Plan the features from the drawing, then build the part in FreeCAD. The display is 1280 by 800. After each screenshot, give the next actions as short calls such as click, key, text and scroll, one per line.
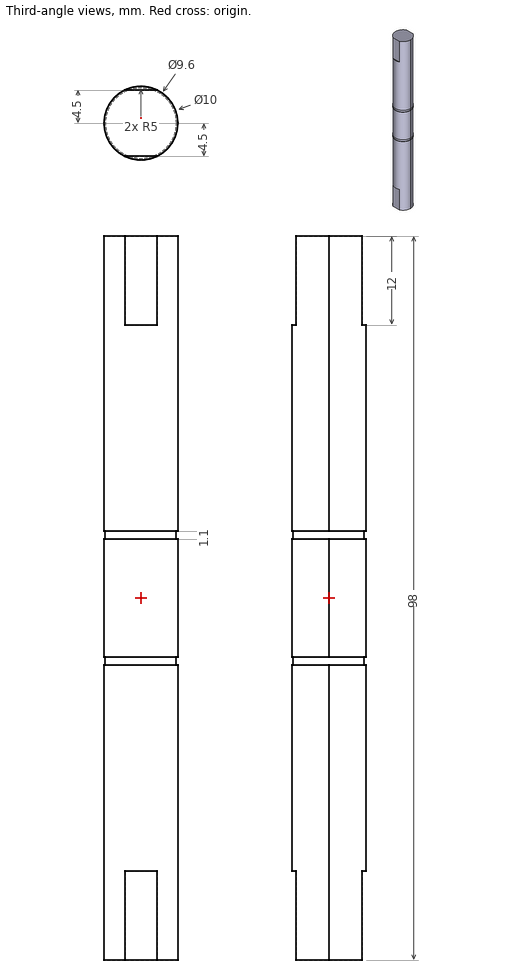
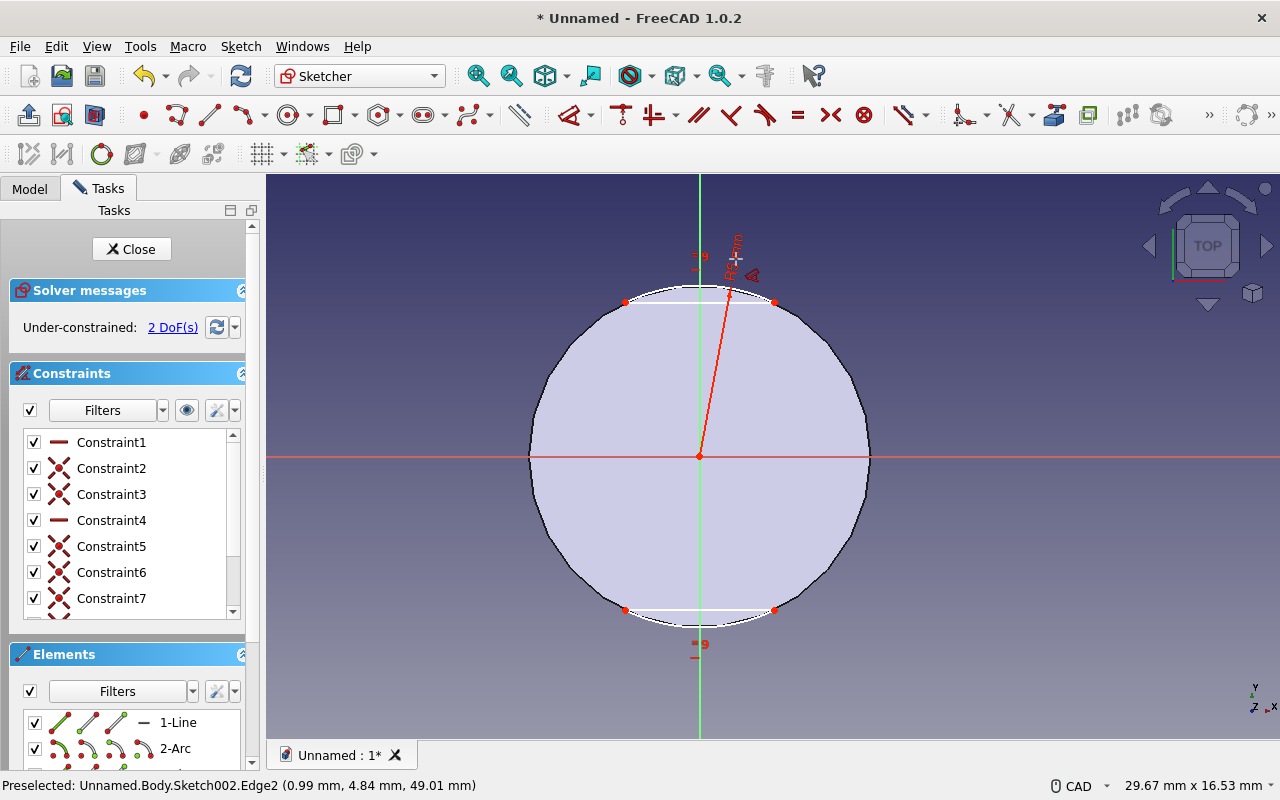
click(625, 303)
click(591, 380)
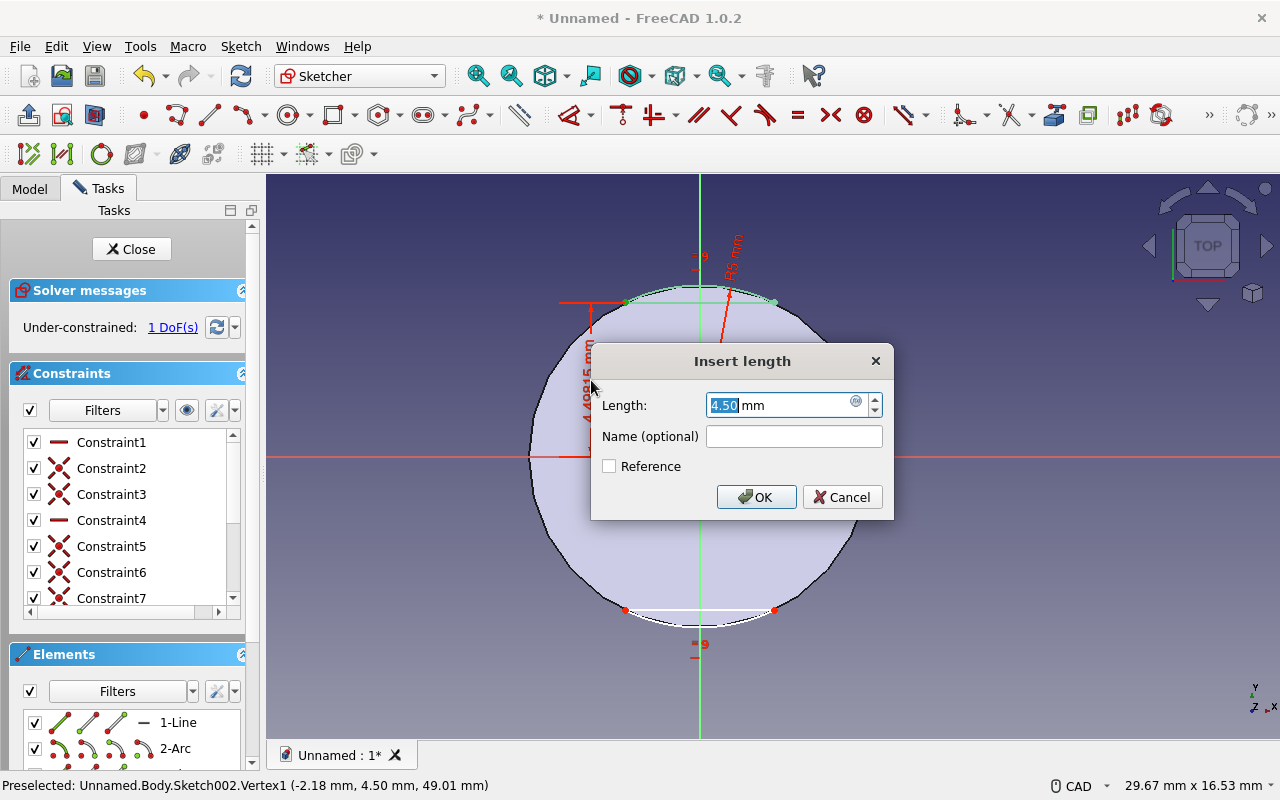
text(4.5)
key(Return)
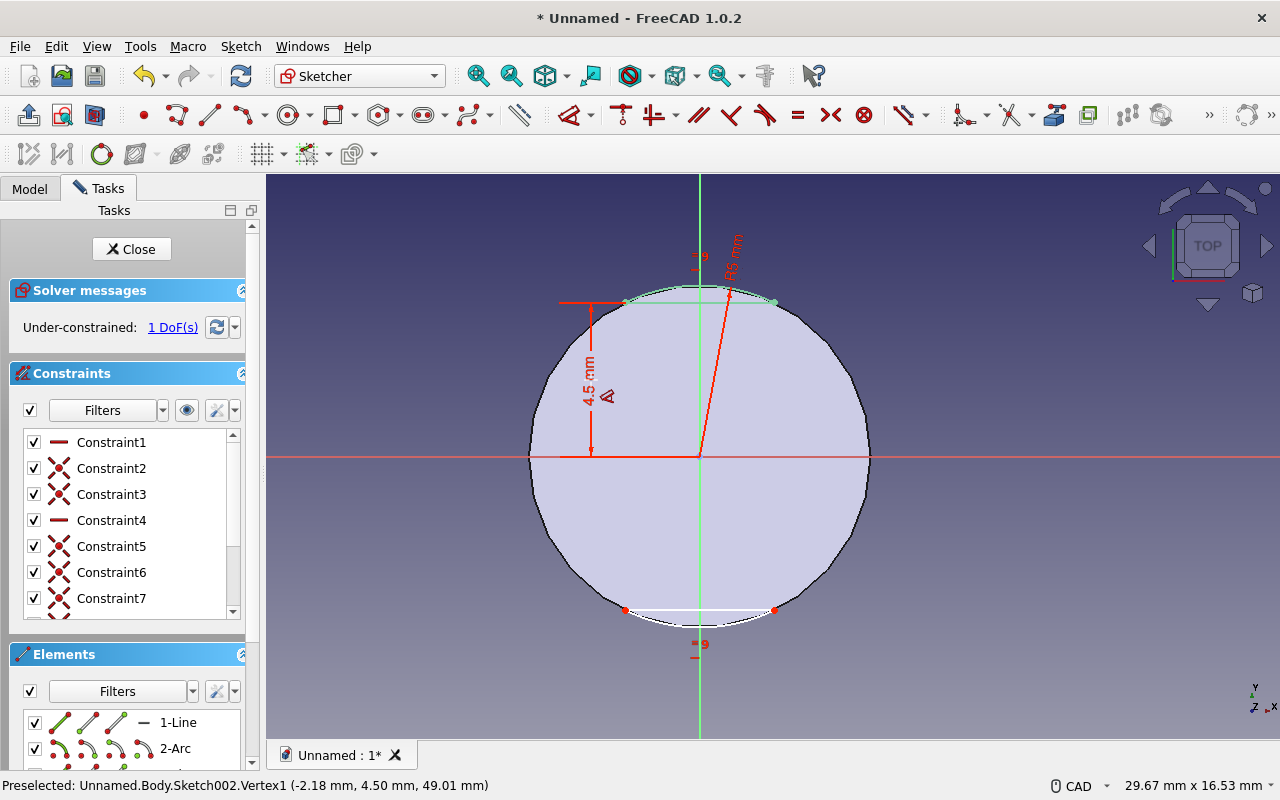
click(774, 610)
click(808, 533)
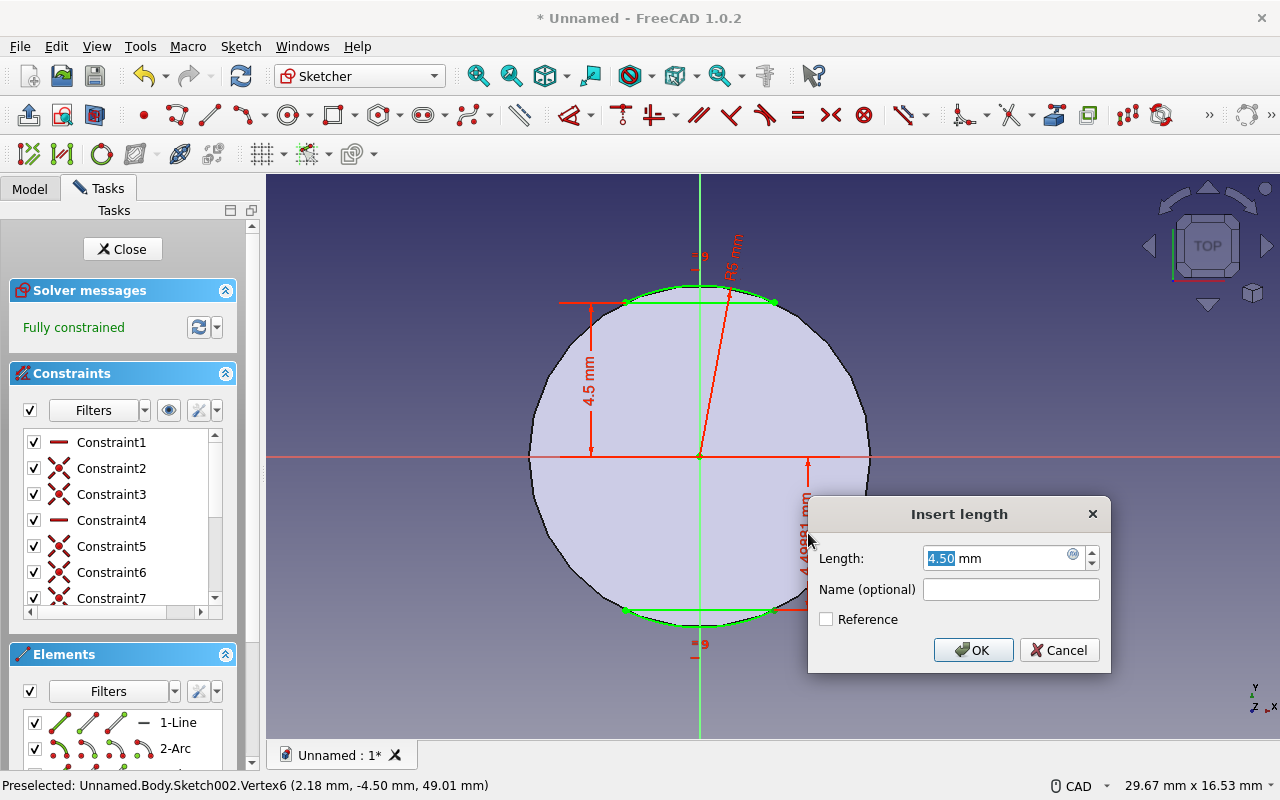
text(4.5)
key(Return)
key(Escape)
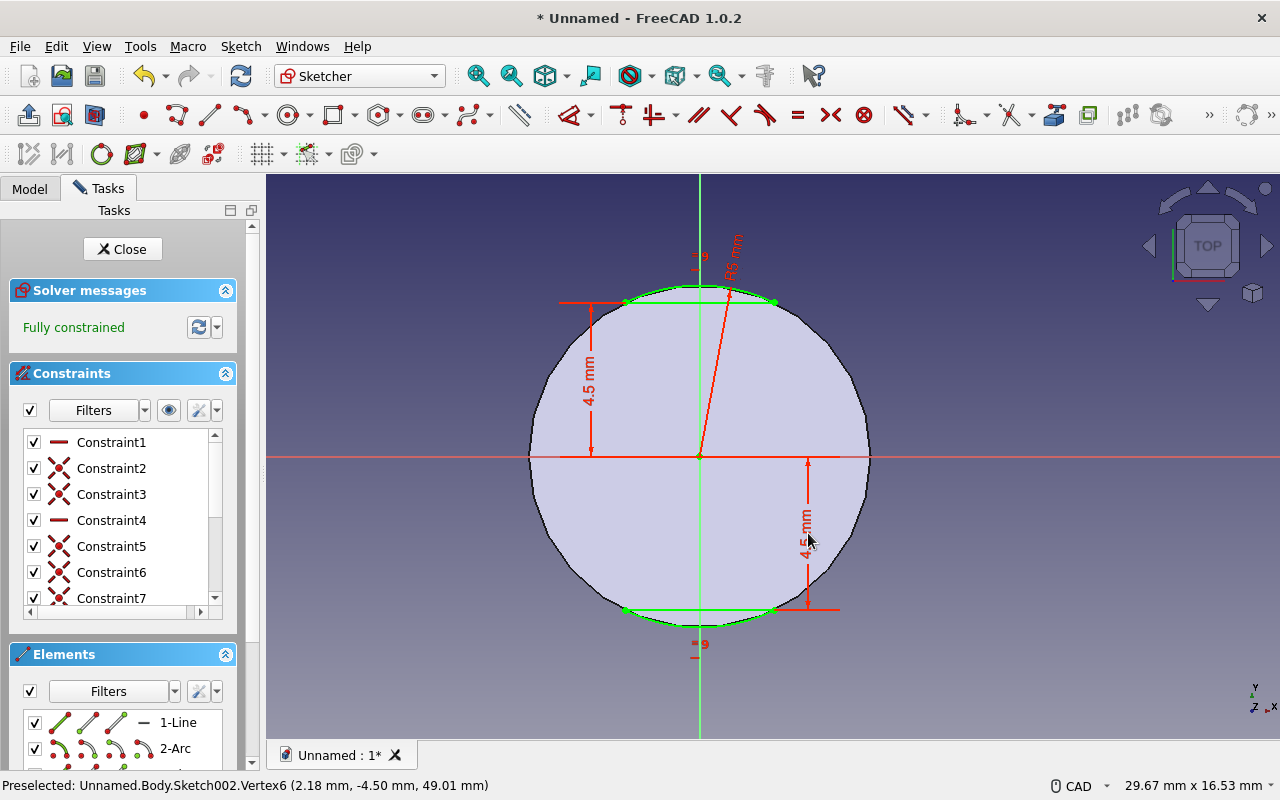
click(123, 249)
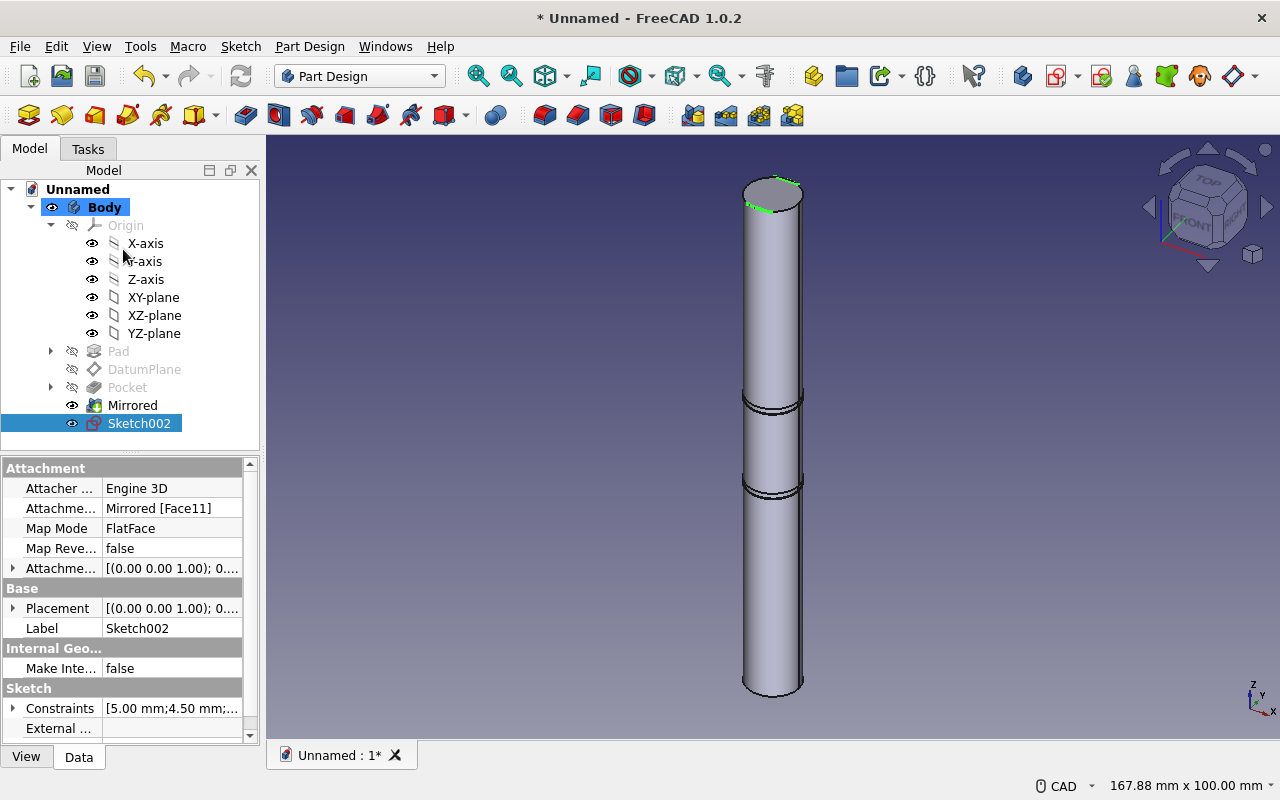
click(246, 116)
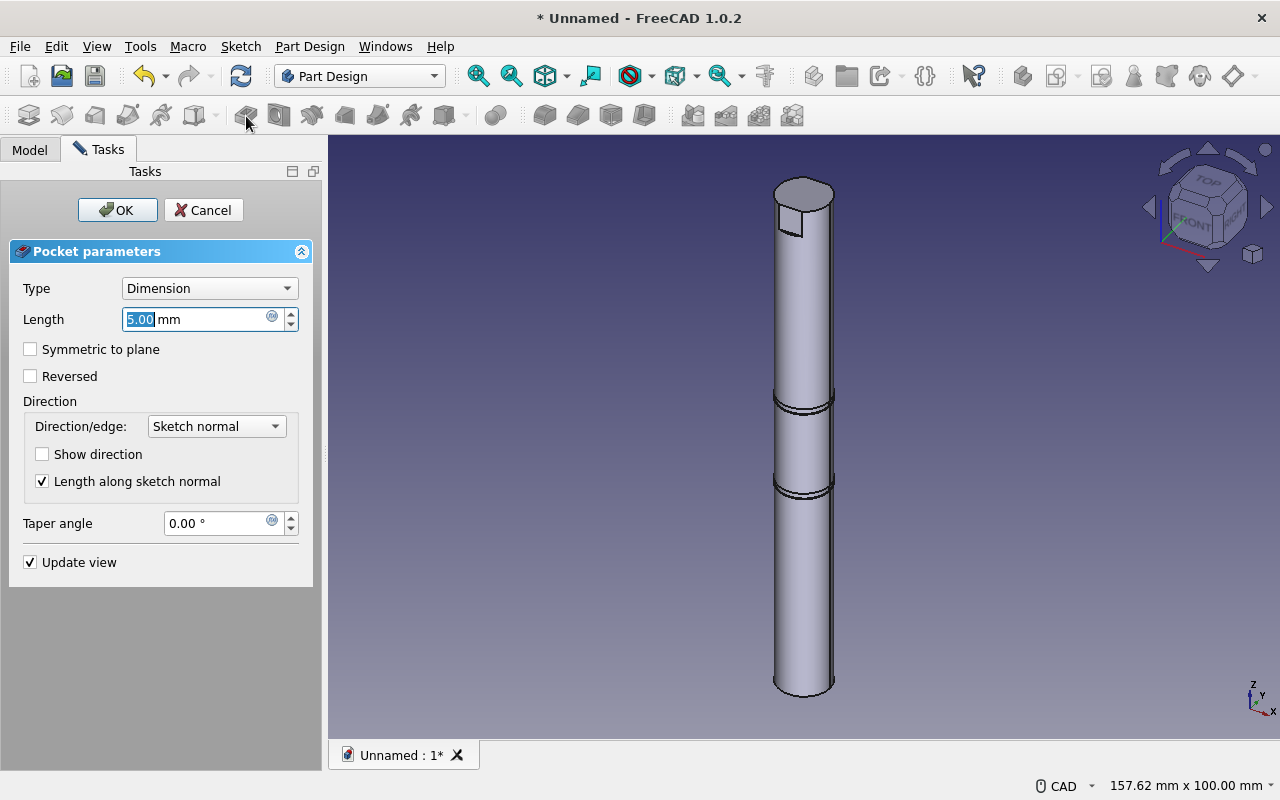
text(12)
key(Tab)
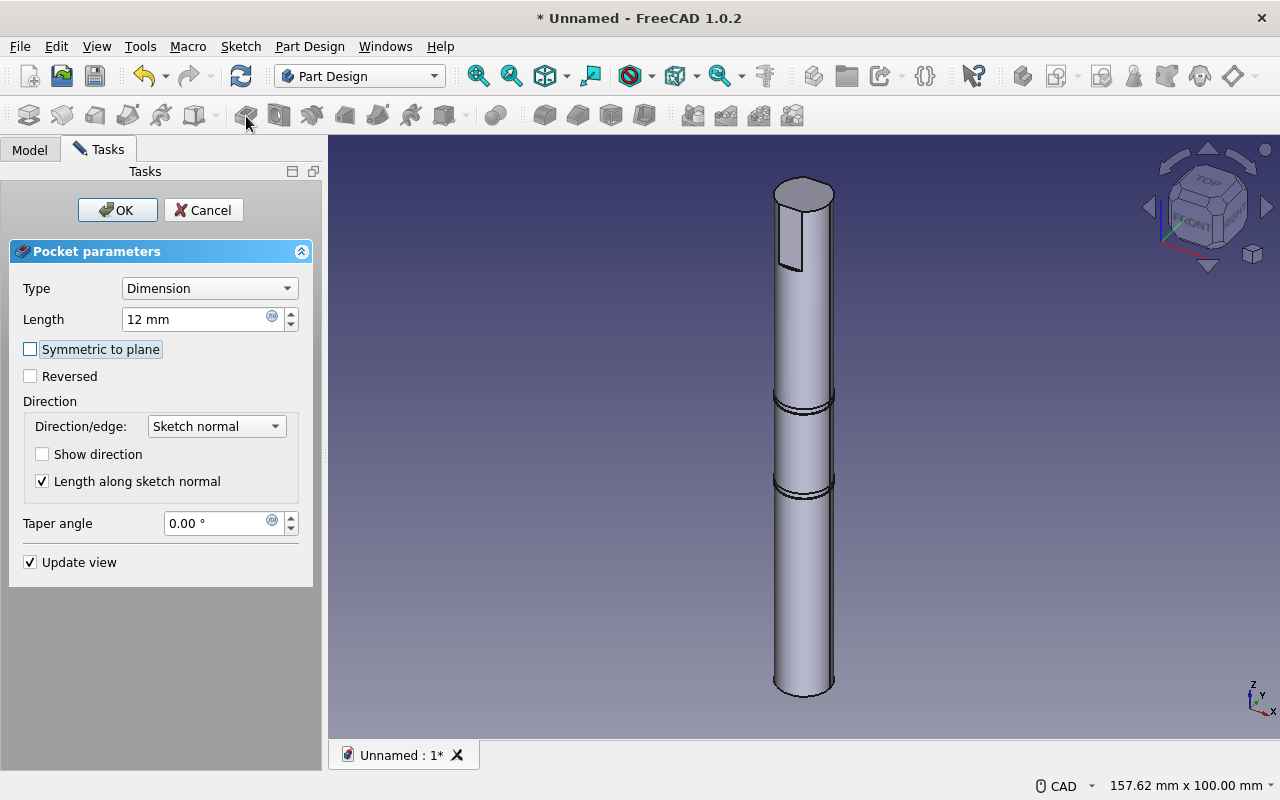
click(118, 210)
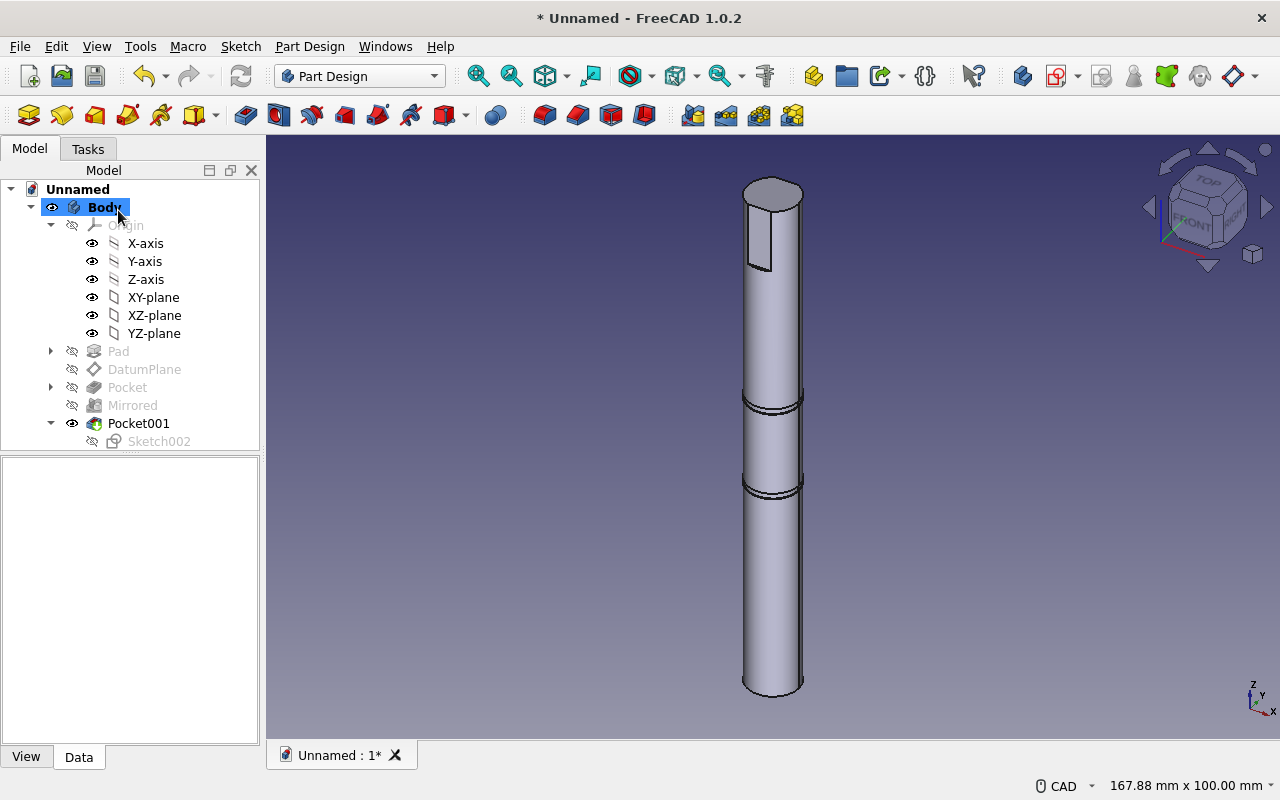
click(117, 423)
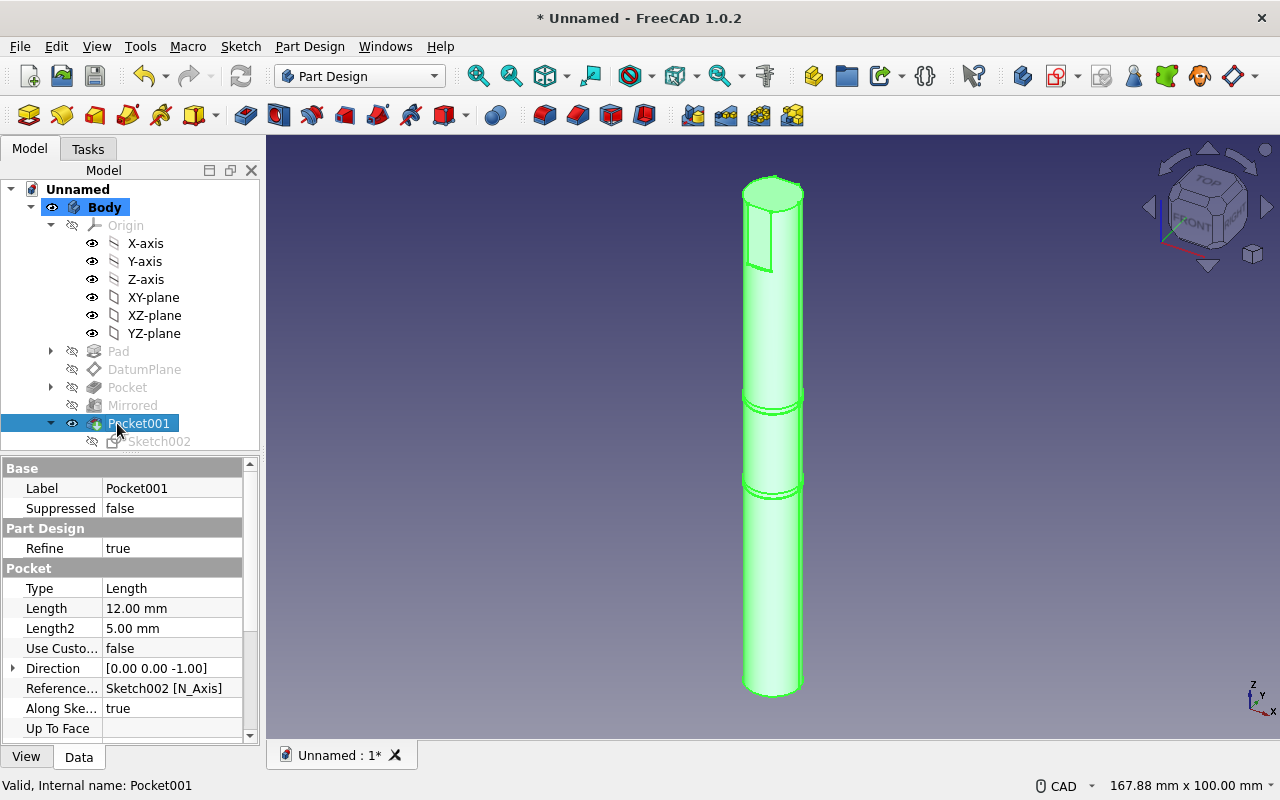
click(693, 116)